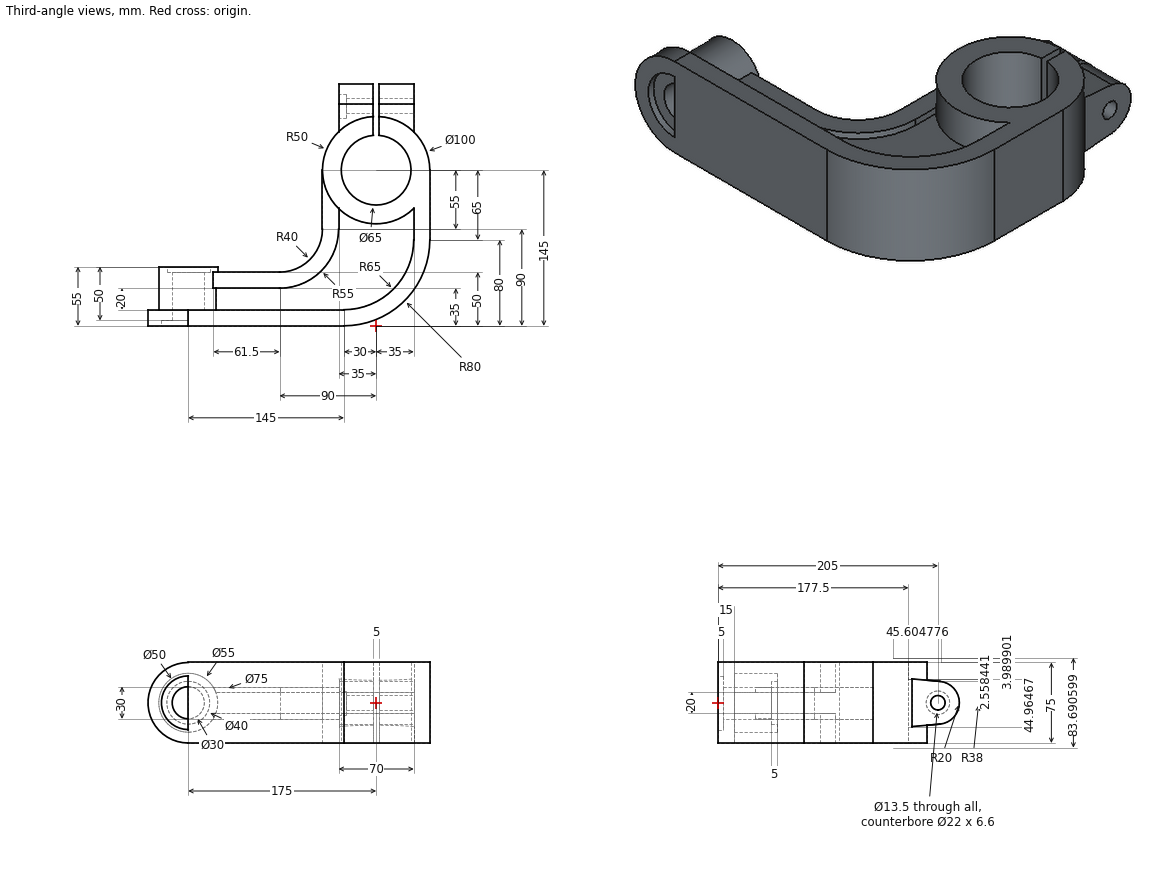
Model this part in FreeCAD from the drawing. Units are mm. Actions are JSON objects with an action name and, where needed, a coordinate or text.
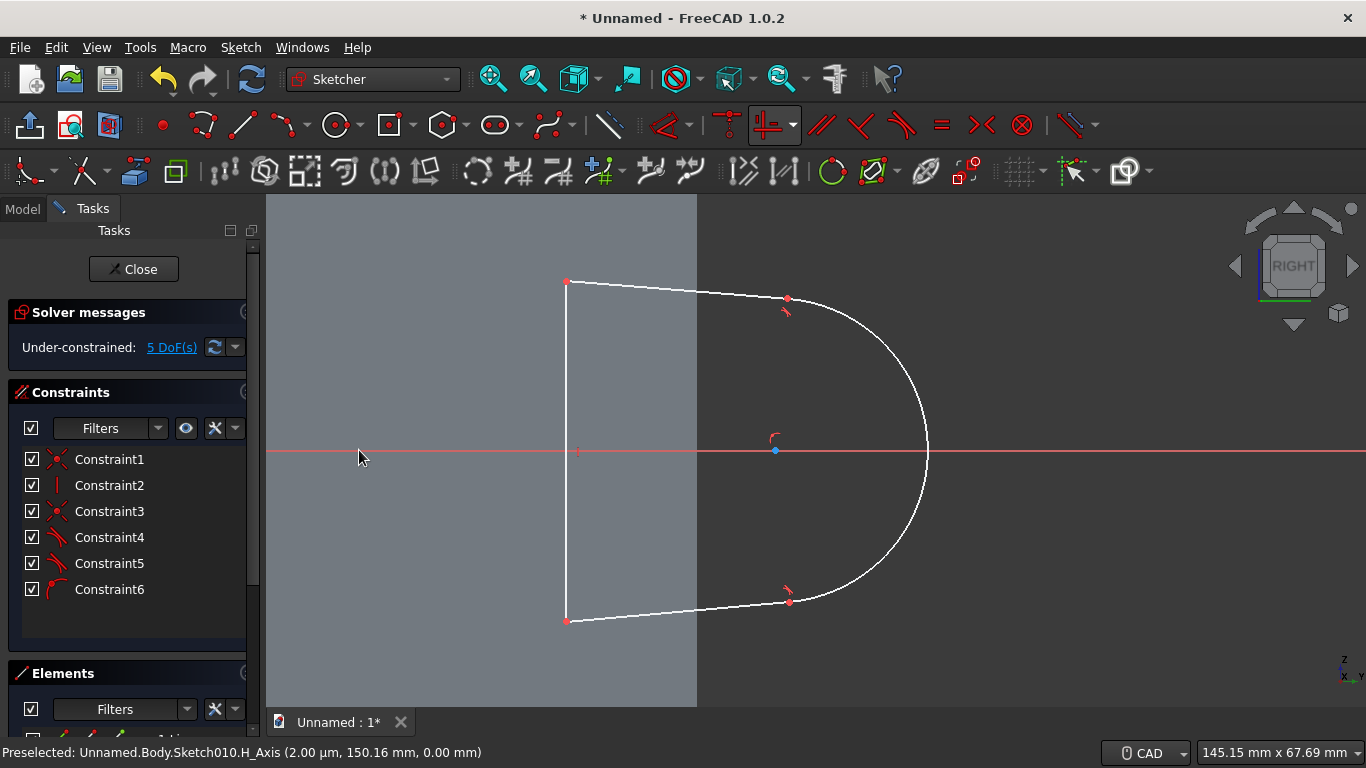
{"action": "left_click", "coordinate": [664, 126]}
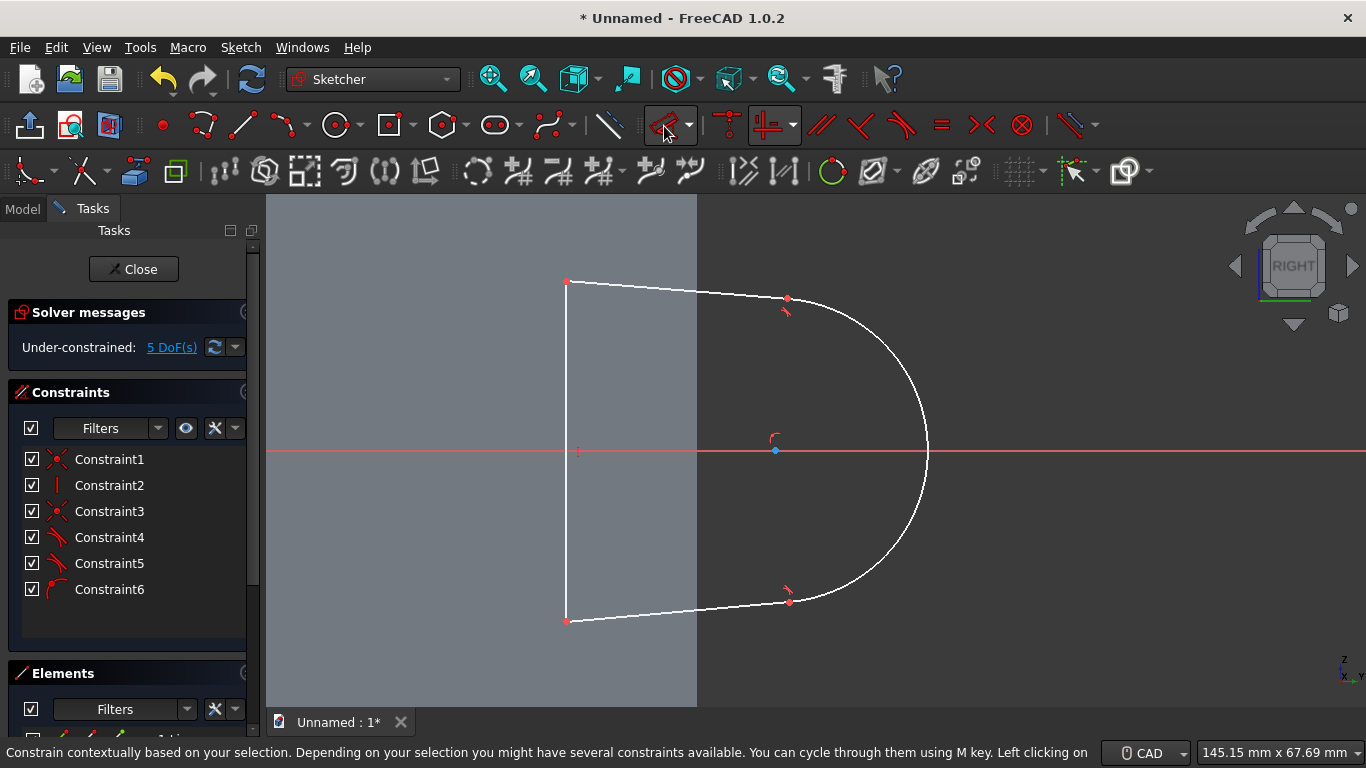
{"action": "left_click", "coordinate": [902, 535]}
{"action": "left_click", "coordinate": [929, 553]}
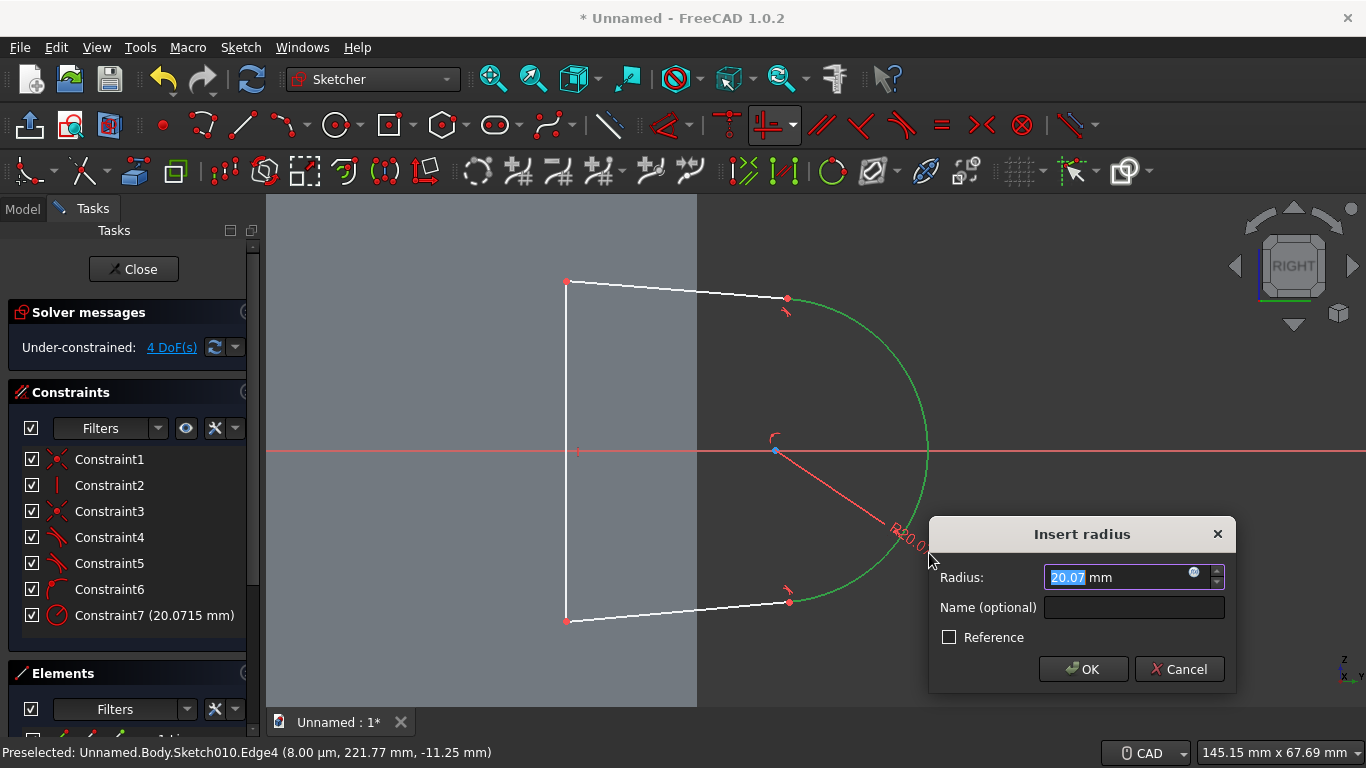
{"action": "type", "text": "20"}
{"action": "key", "text": "Return"}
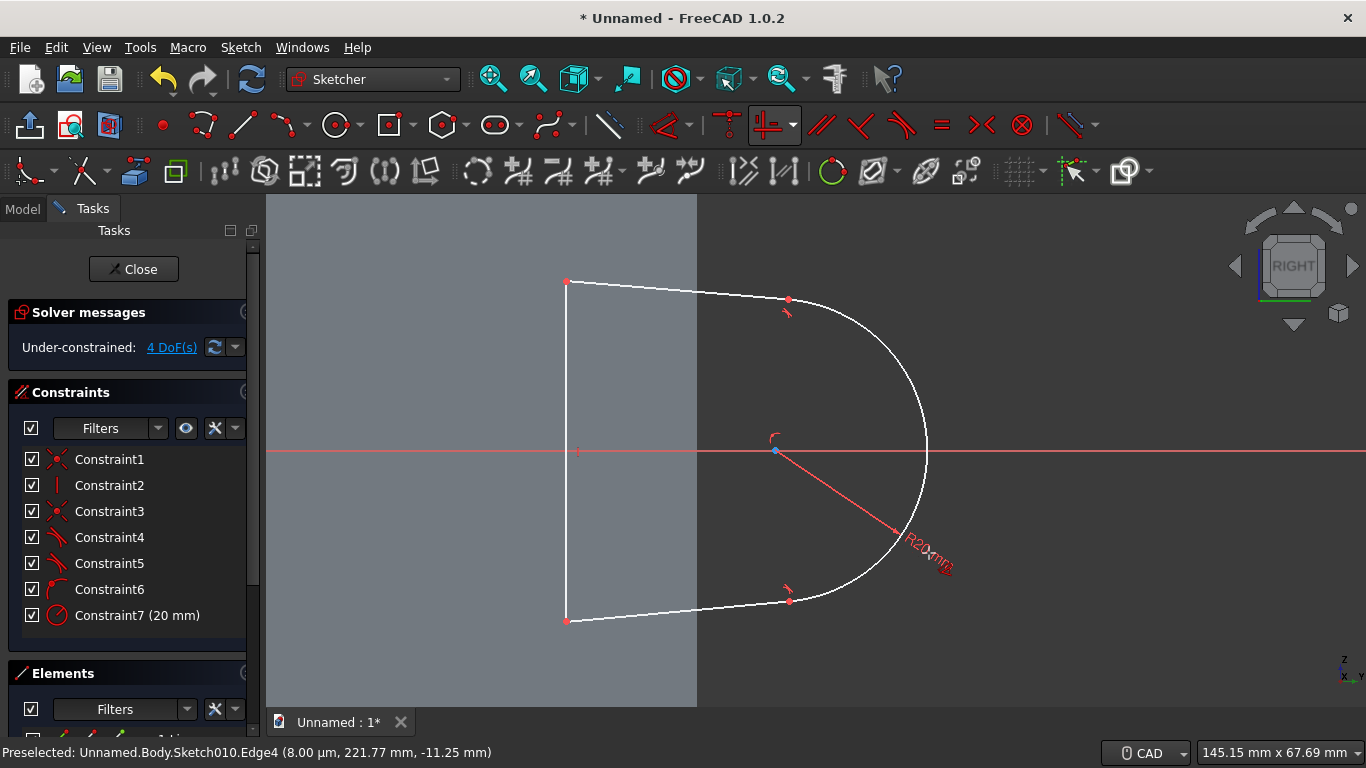
{"action": "left_click", "coordinate": [776, 450]}
{"action": "left_click", "coordinate": [535, 484]}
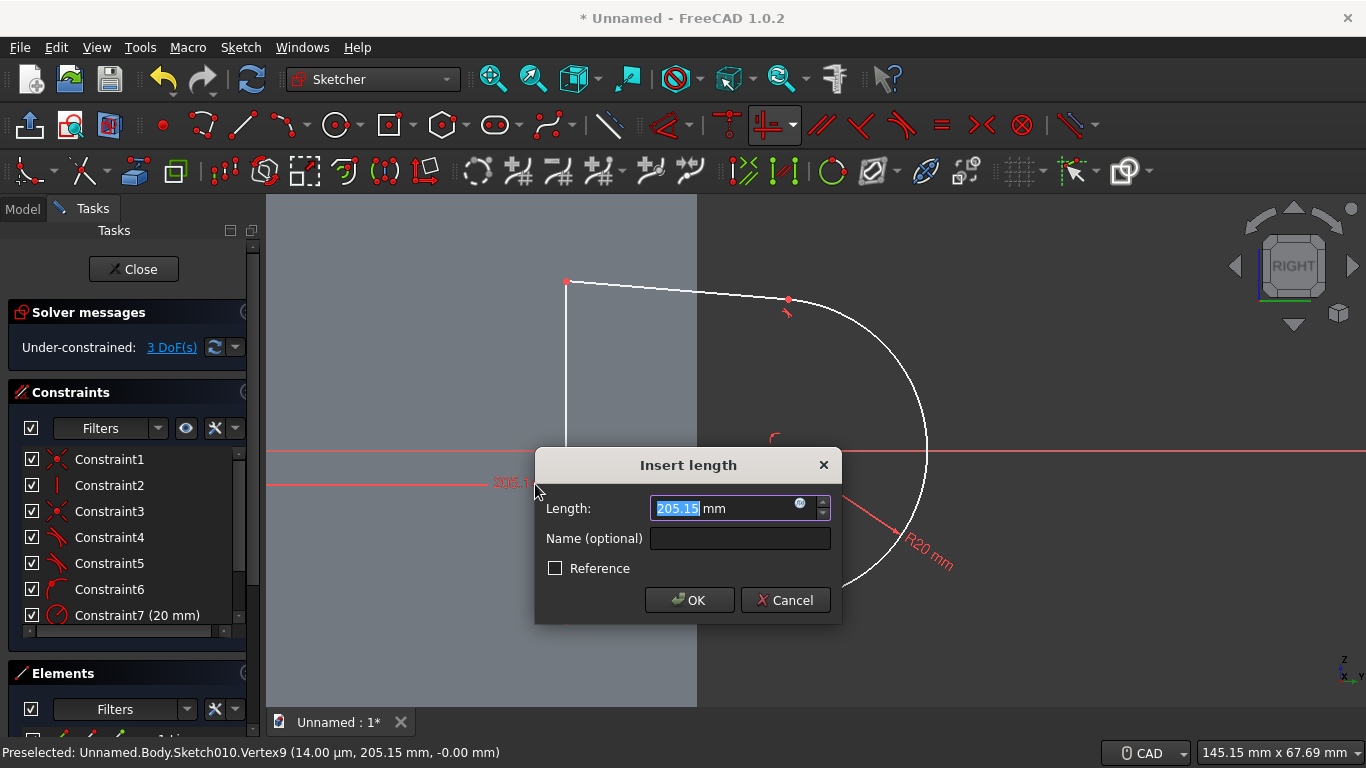
{"action": "type", "text": "205"}
{"action": "key", "text": "Return"}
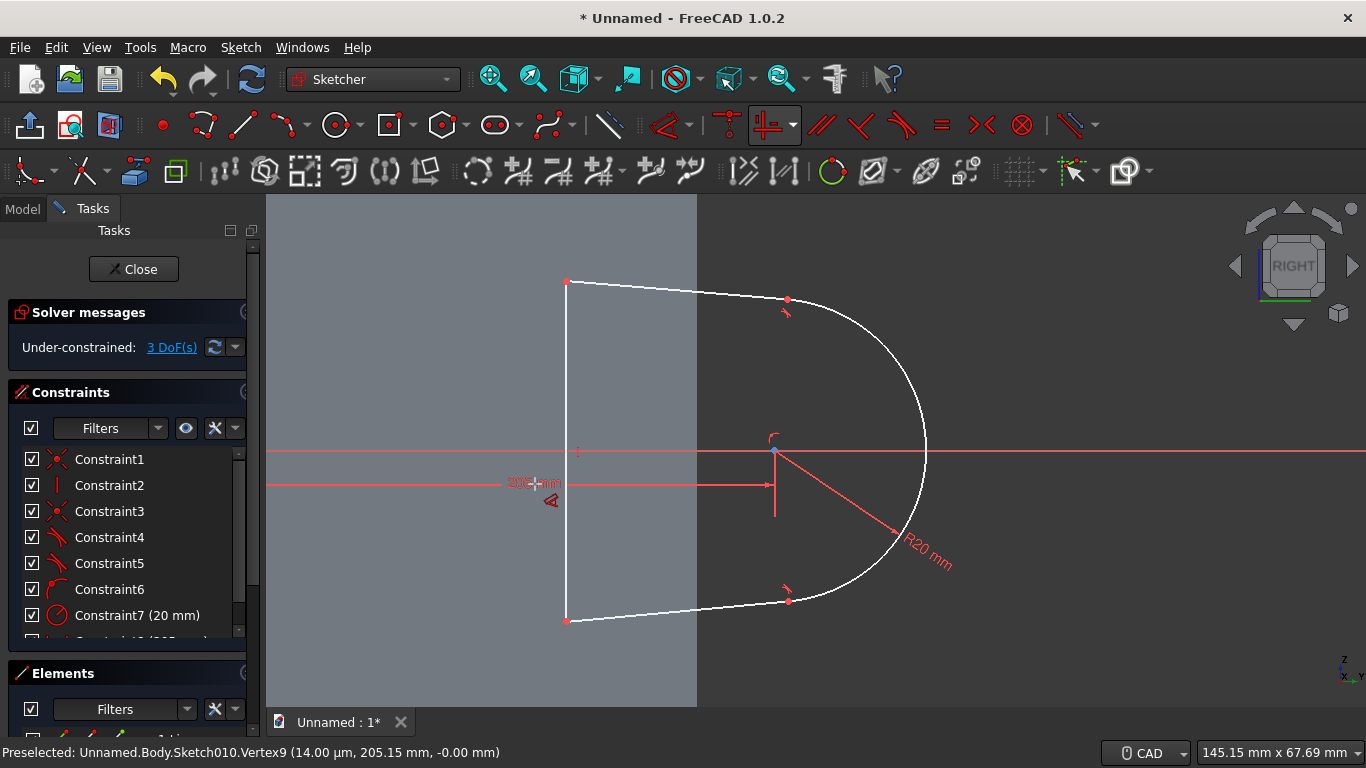
{"action": "left_click", "coordinate": [566, 281]}
{"action": "left_click", "coordinate": [430, 247]}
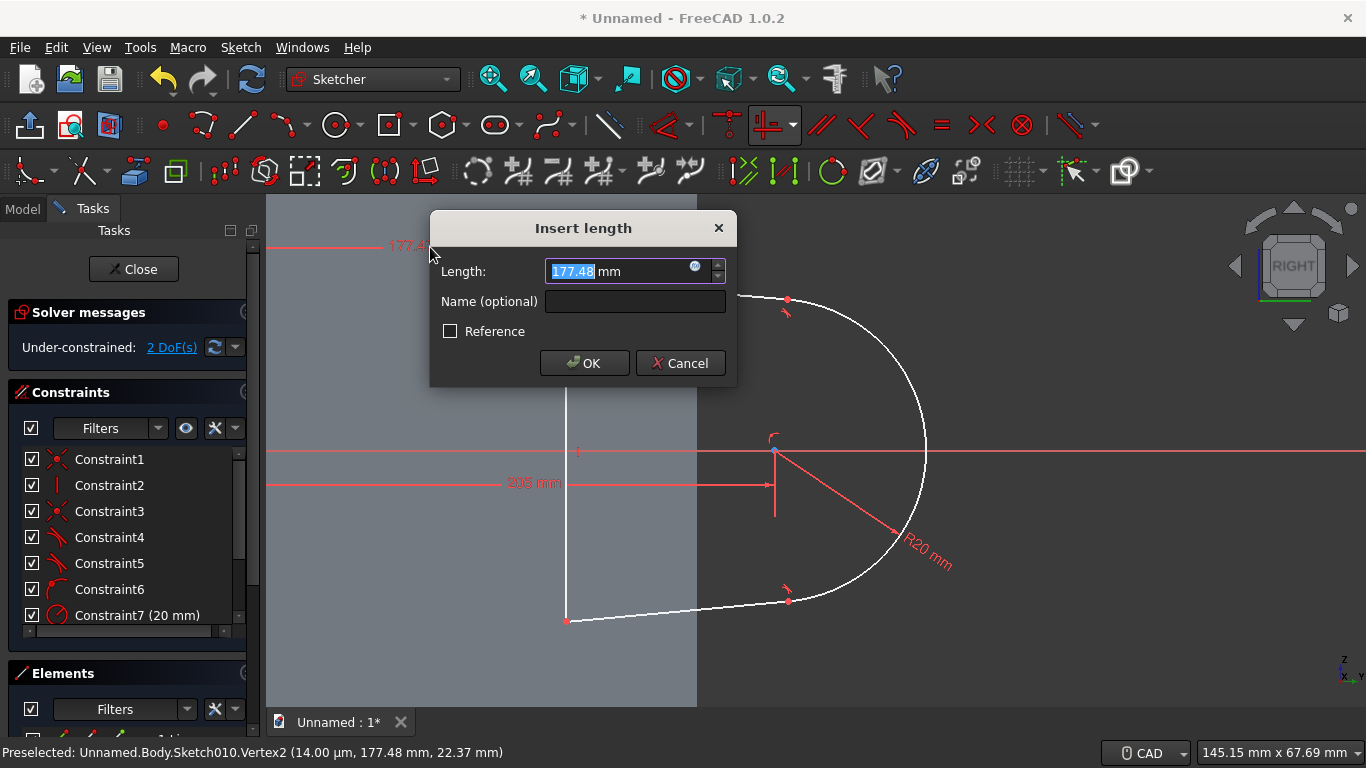
{"action": "type", "text": "177.5"}
{"action": "key", "text": "Return"}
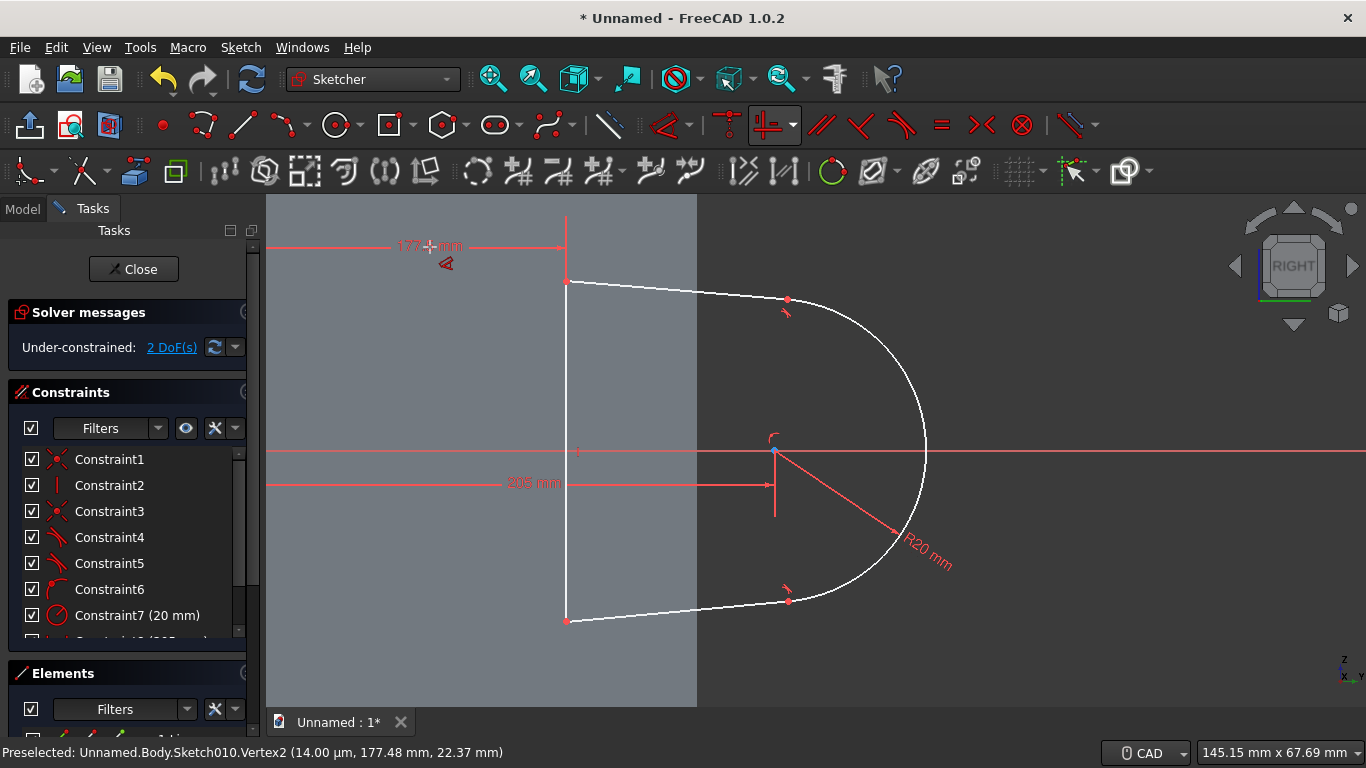
{"action": "left_click", "coordinate": [566, 383]}
{"action": "left_click", "coordinate": [532, 373]}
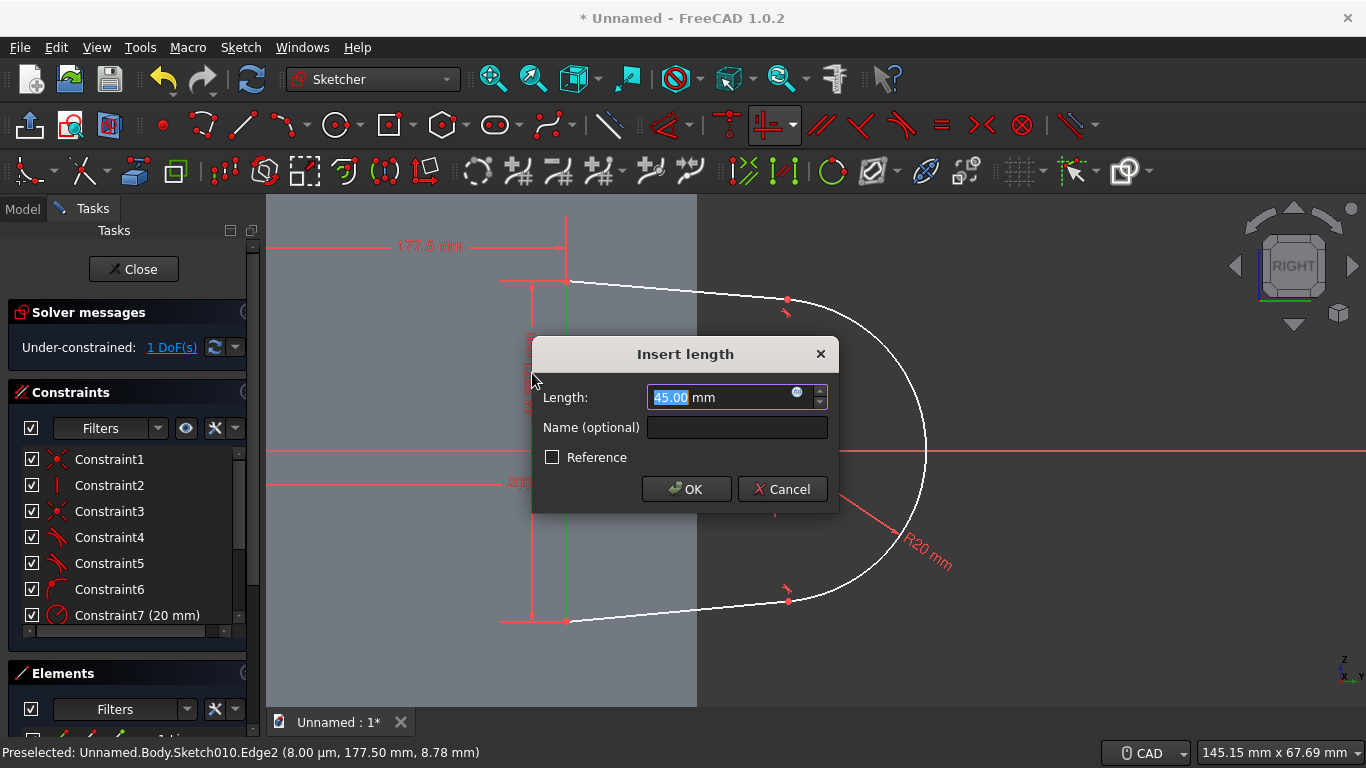
{"action": "type", "text": "44.96467"}
{"action": "key", "text": "Return"}